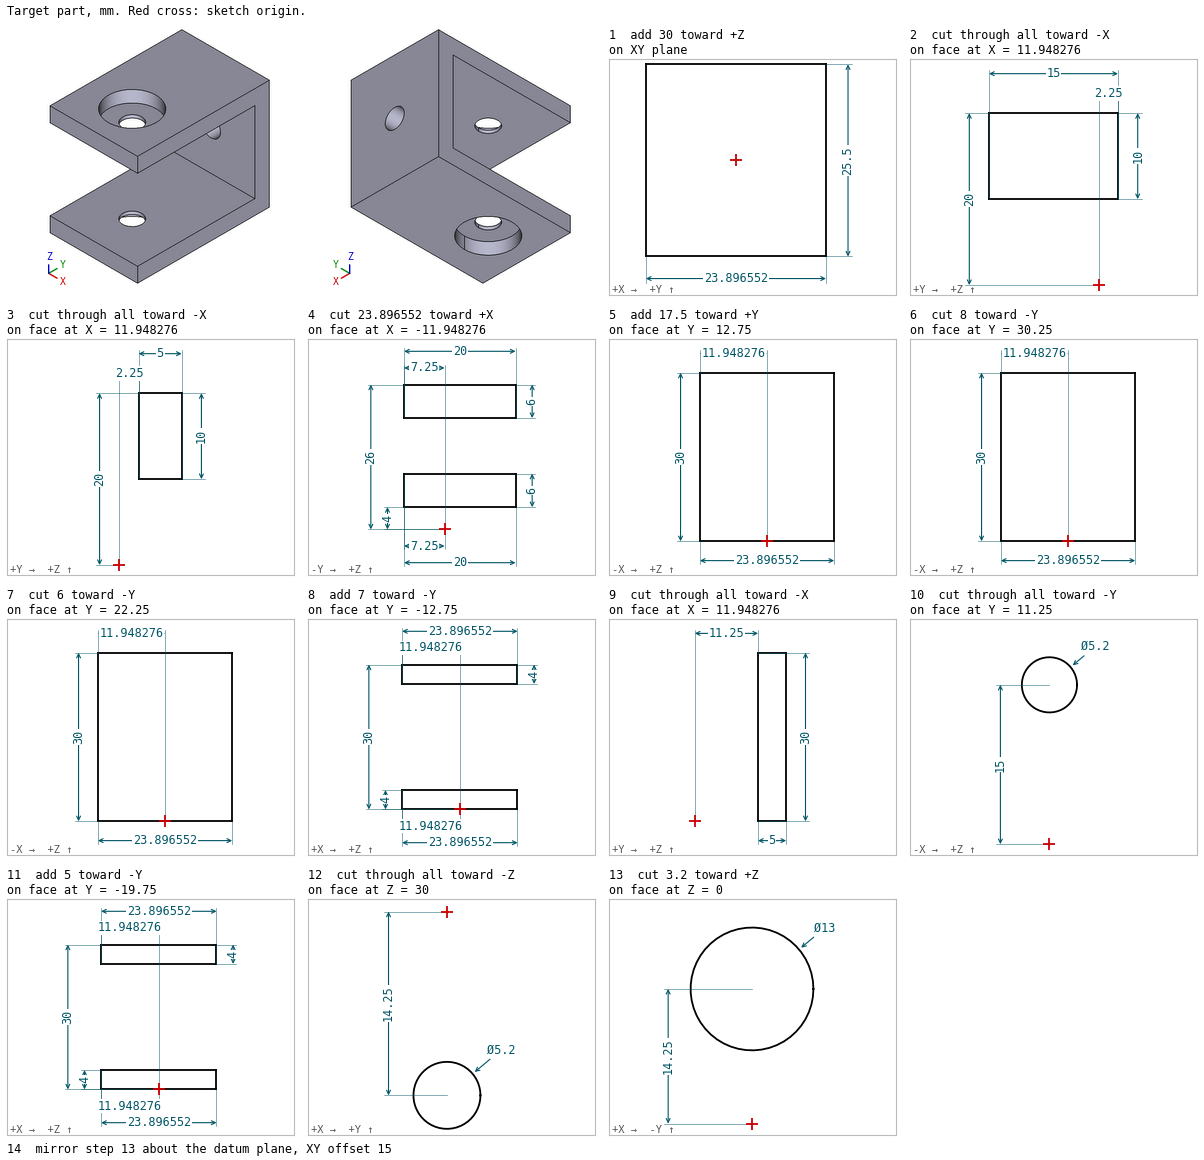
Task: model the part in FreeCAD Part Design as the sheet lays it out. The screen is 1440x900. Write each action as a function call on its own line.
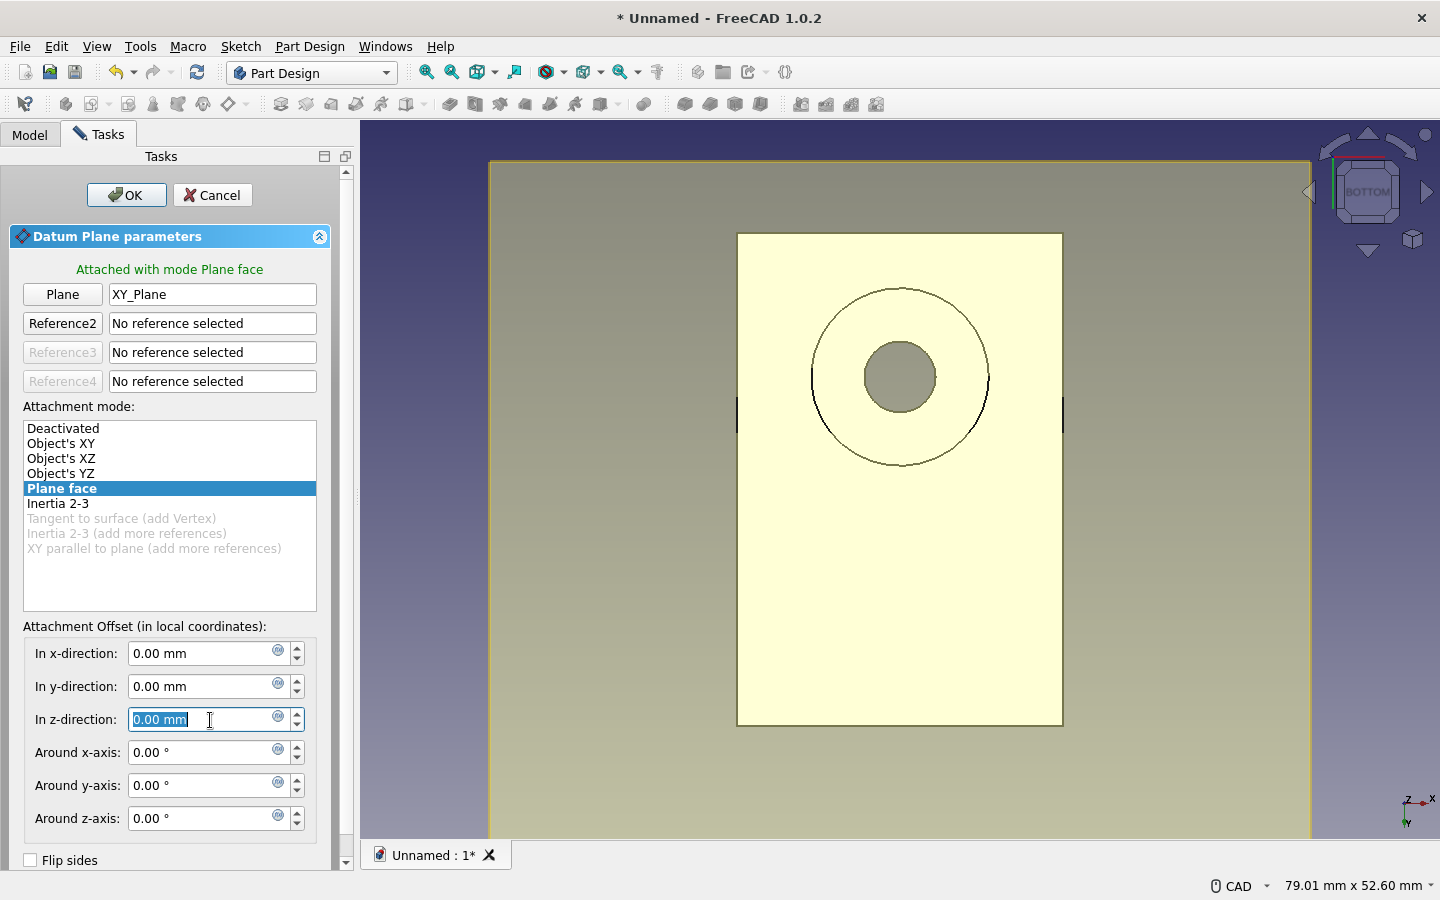
text(15)
key(Tab)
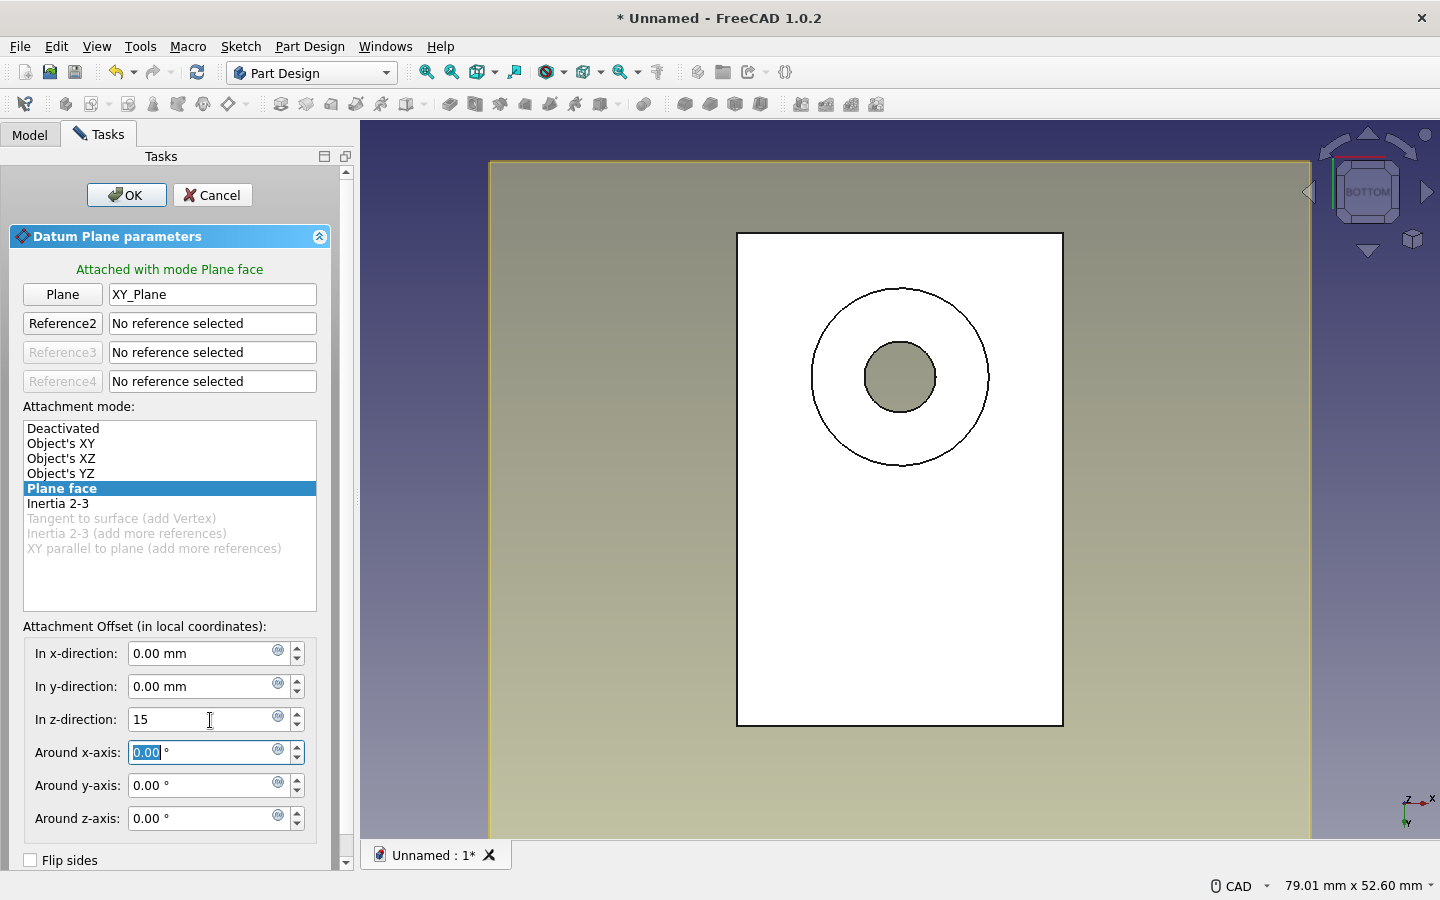
click(127, 195)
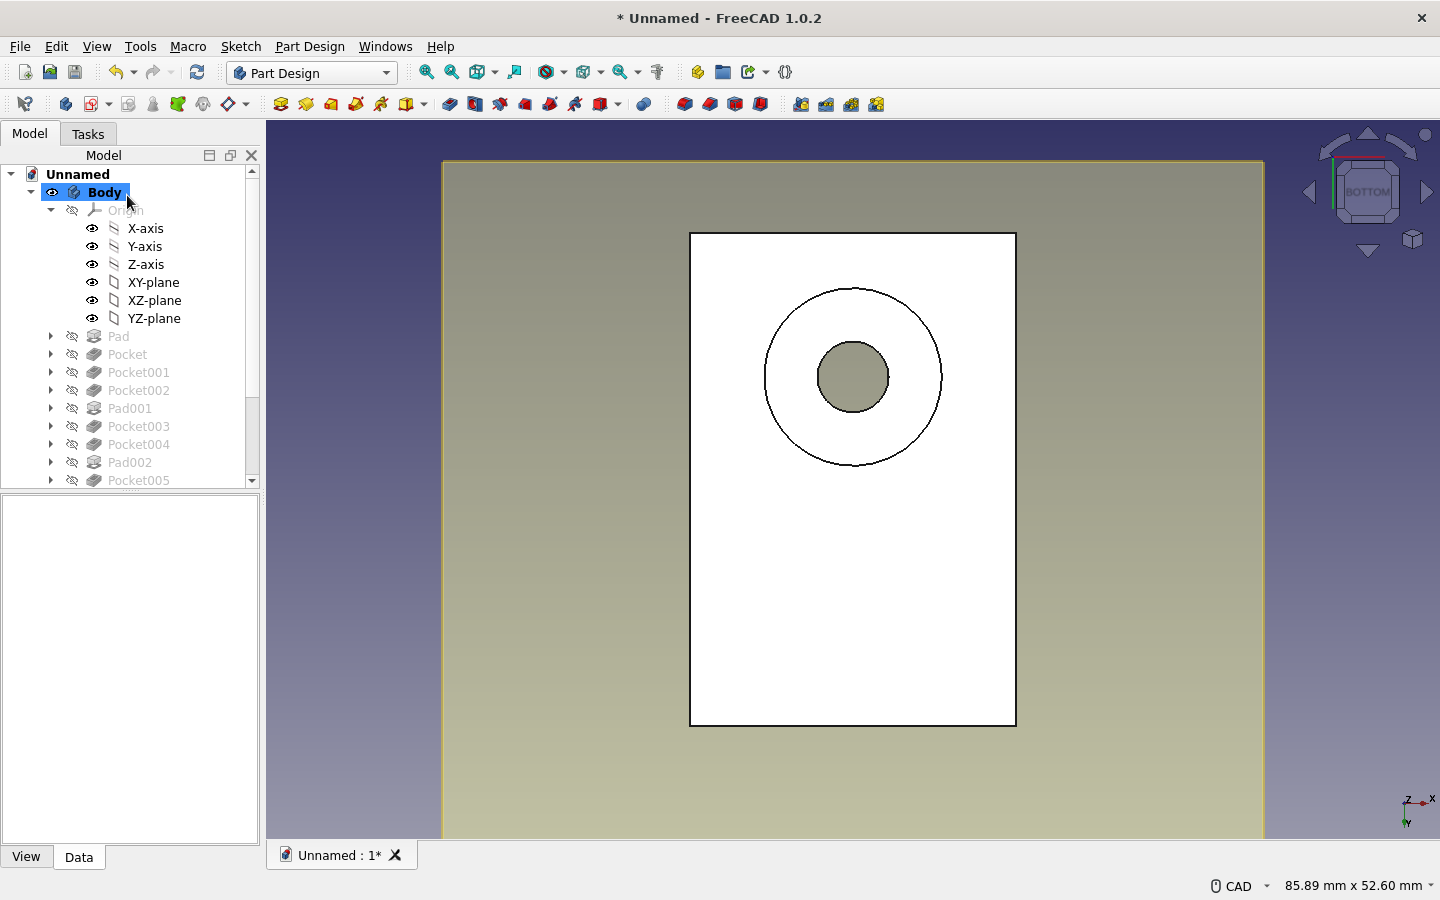
scroll(101, 332, down, 3)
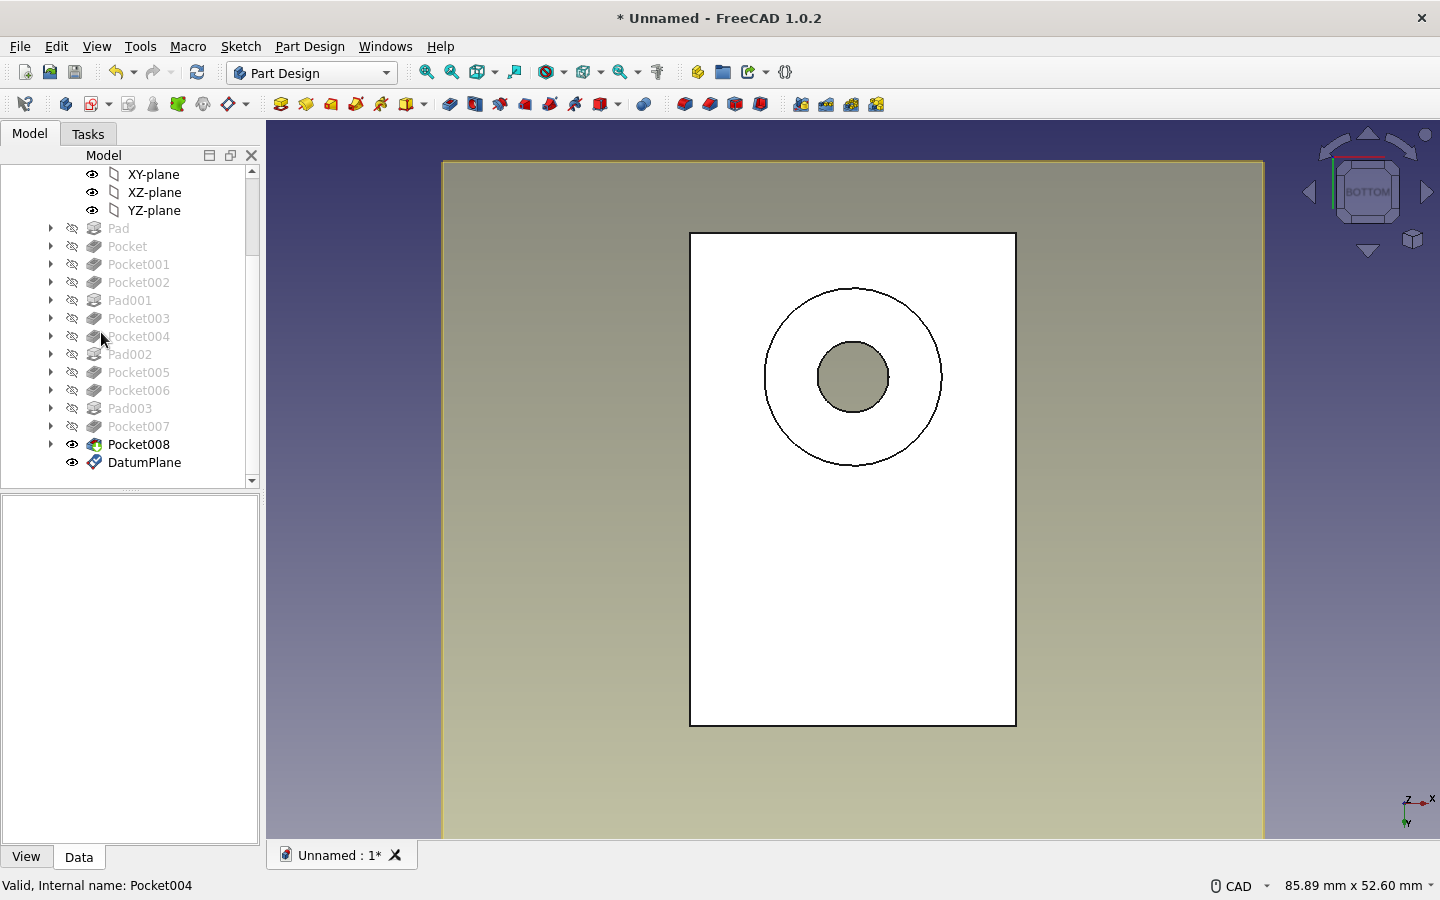
click(117, 444)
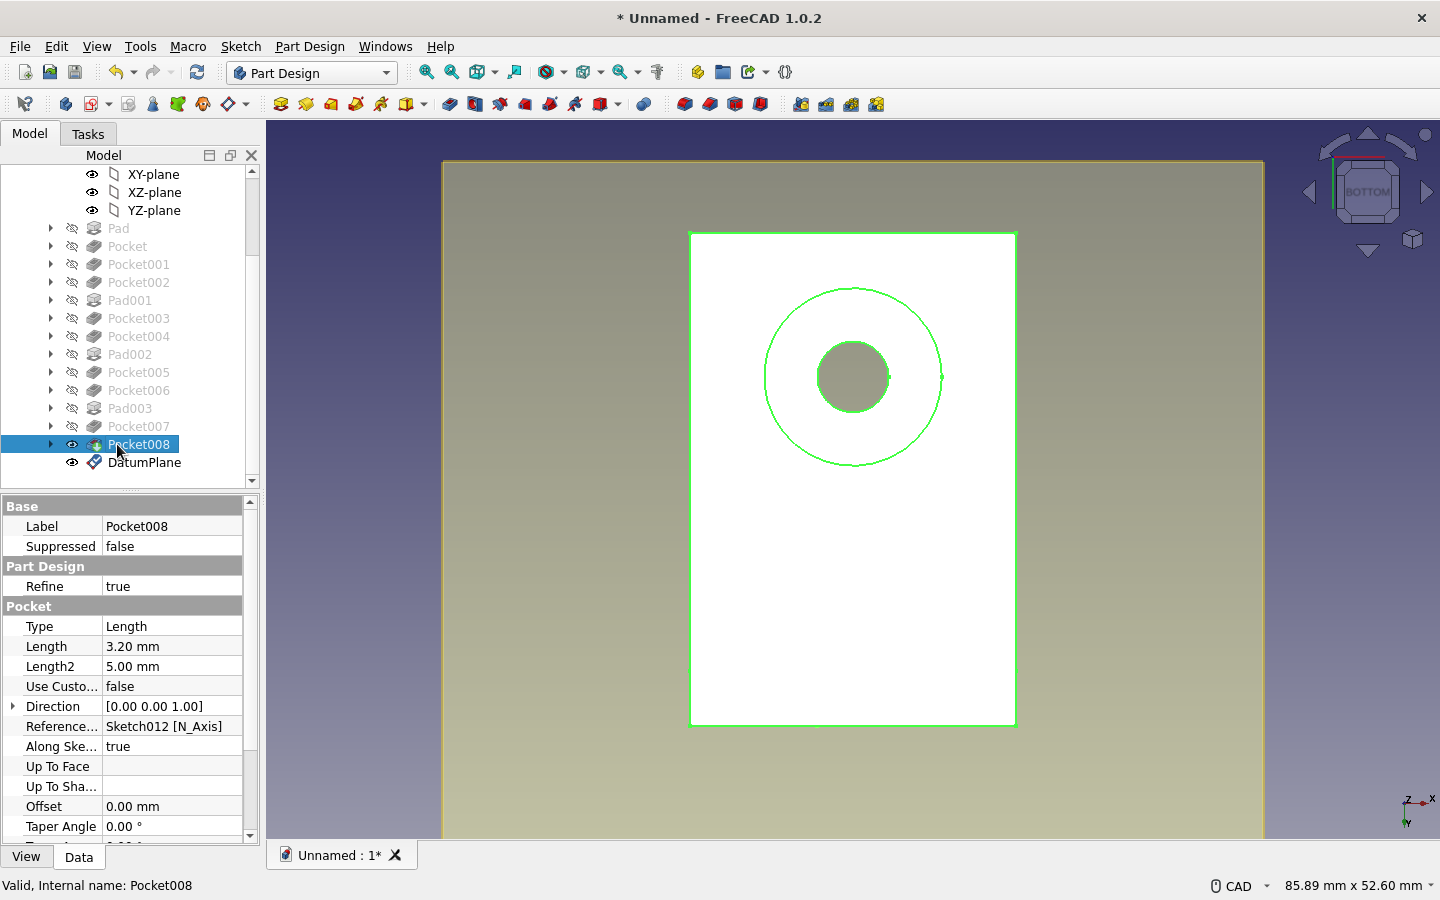
click(801, 104)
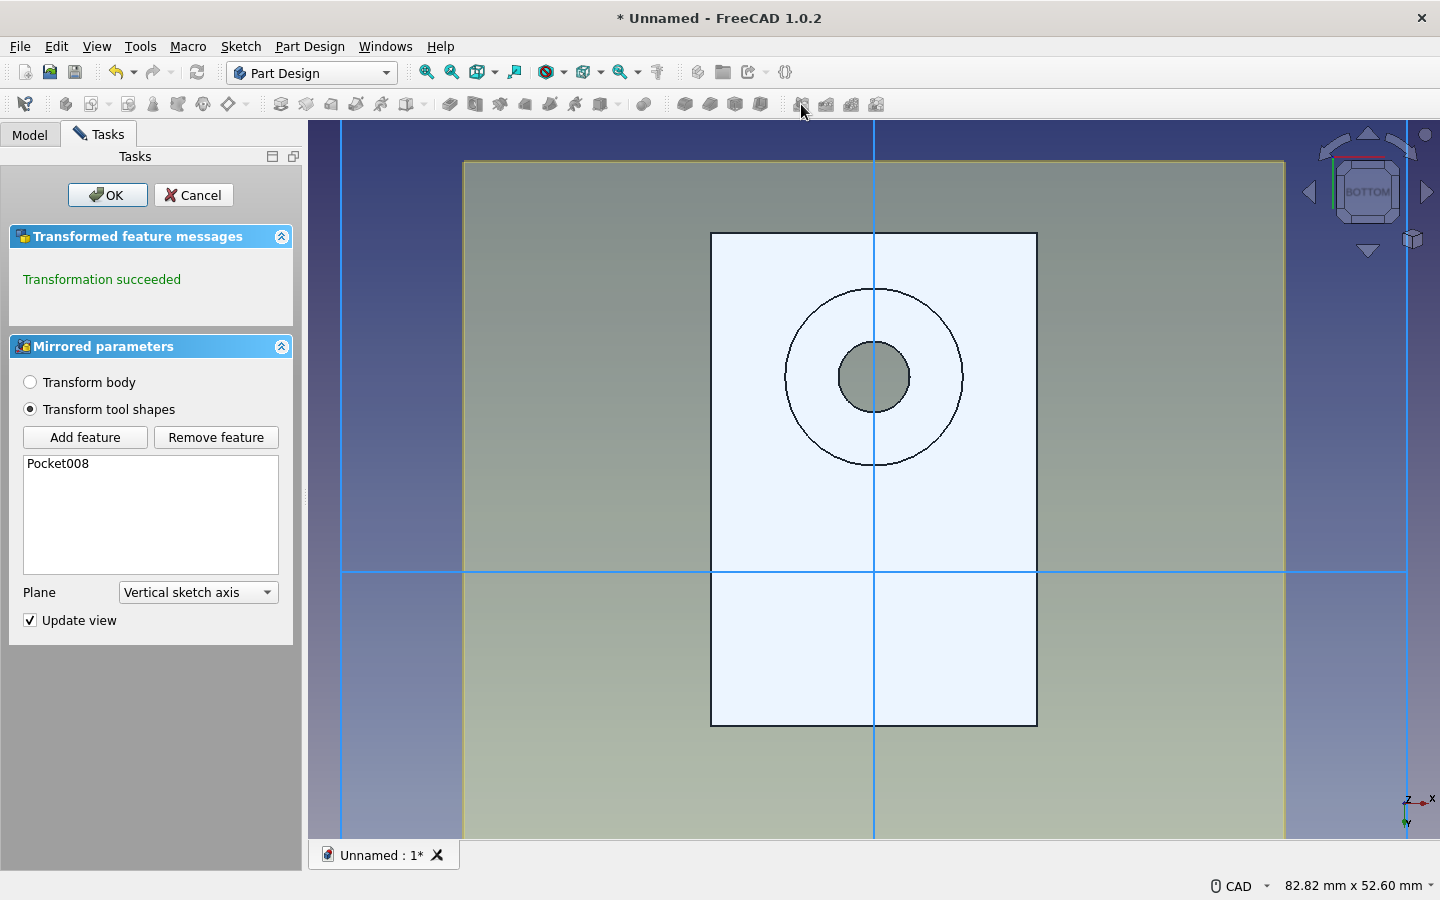
click(199, 592)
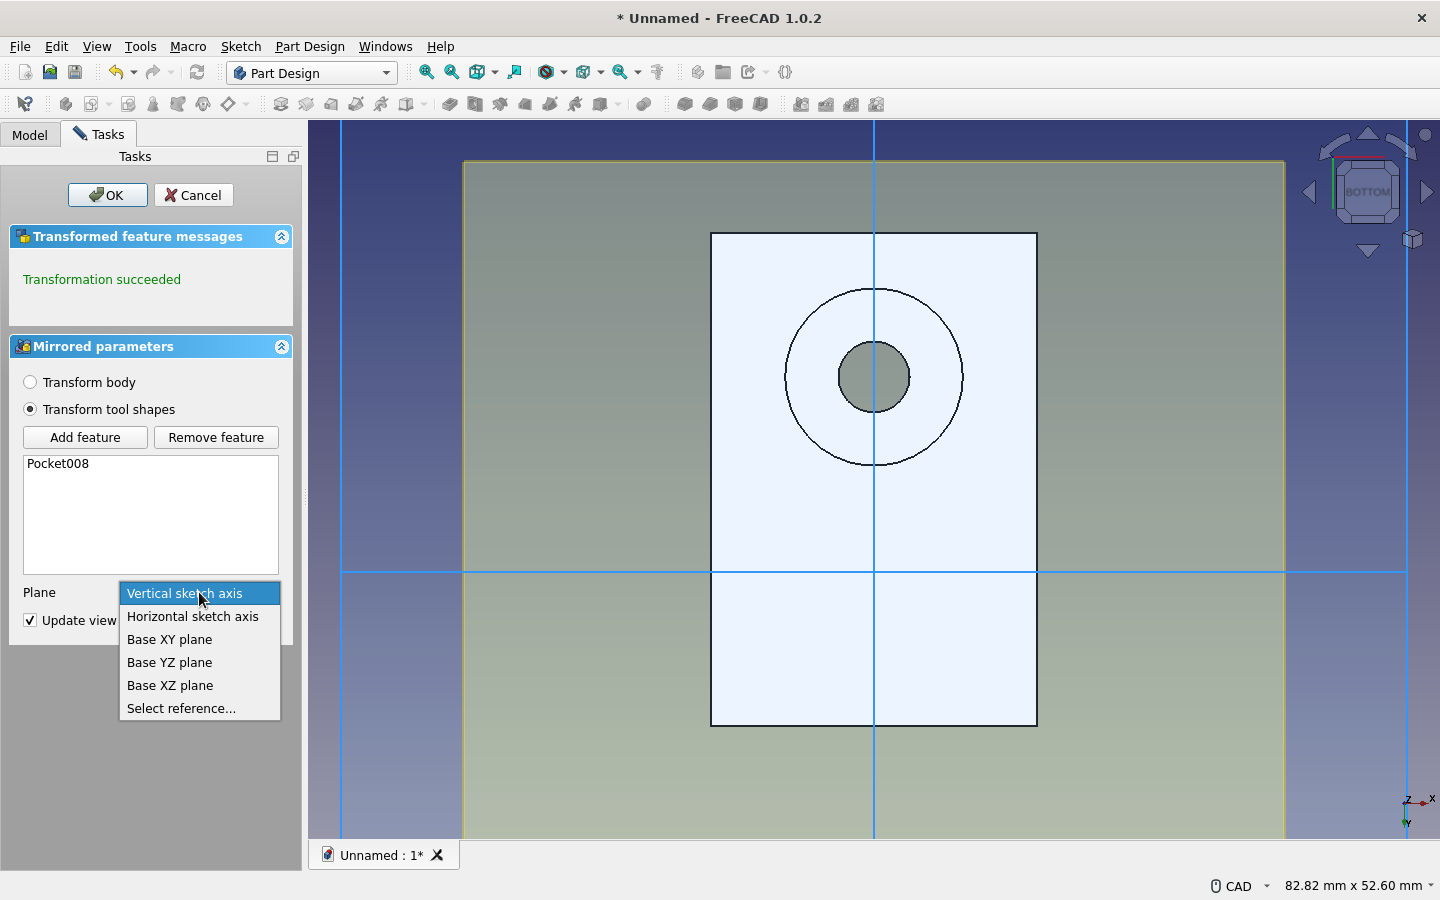
click(198, 708)